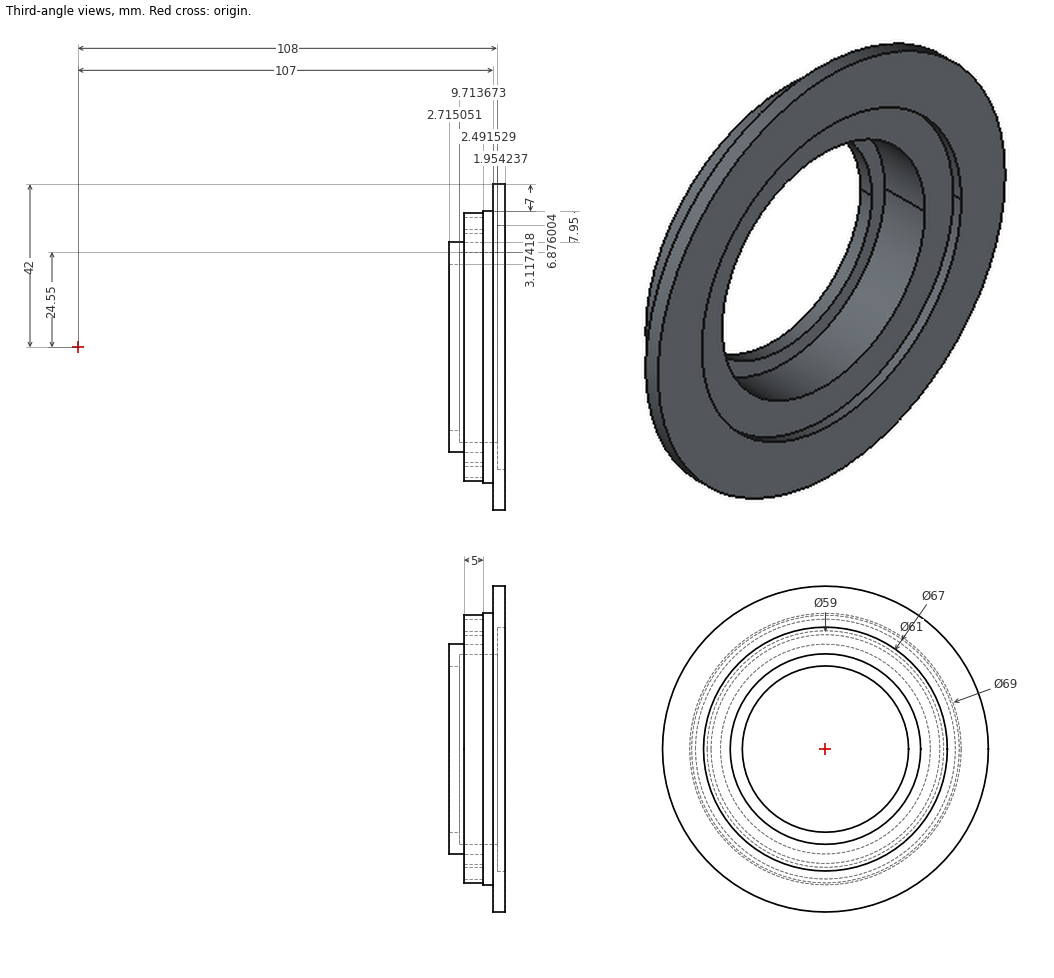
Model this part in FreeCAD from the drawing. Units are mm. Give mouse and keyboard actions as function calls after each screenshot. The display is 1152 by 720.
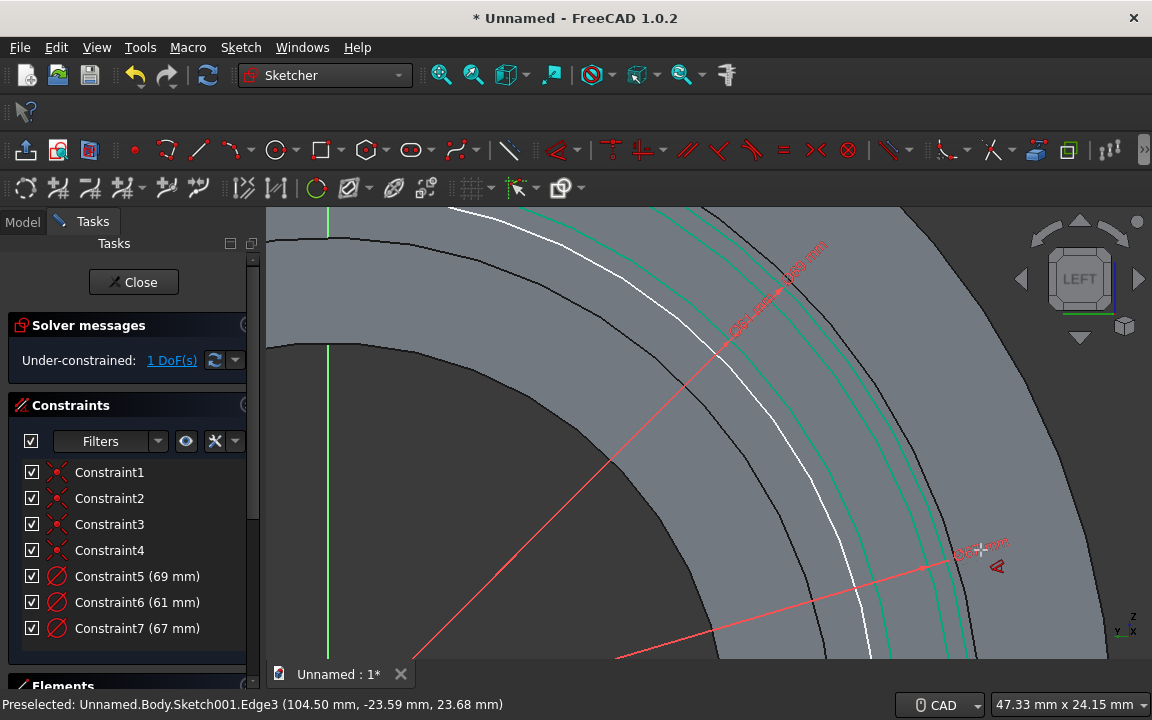
click(716, 353)
click(909, 571)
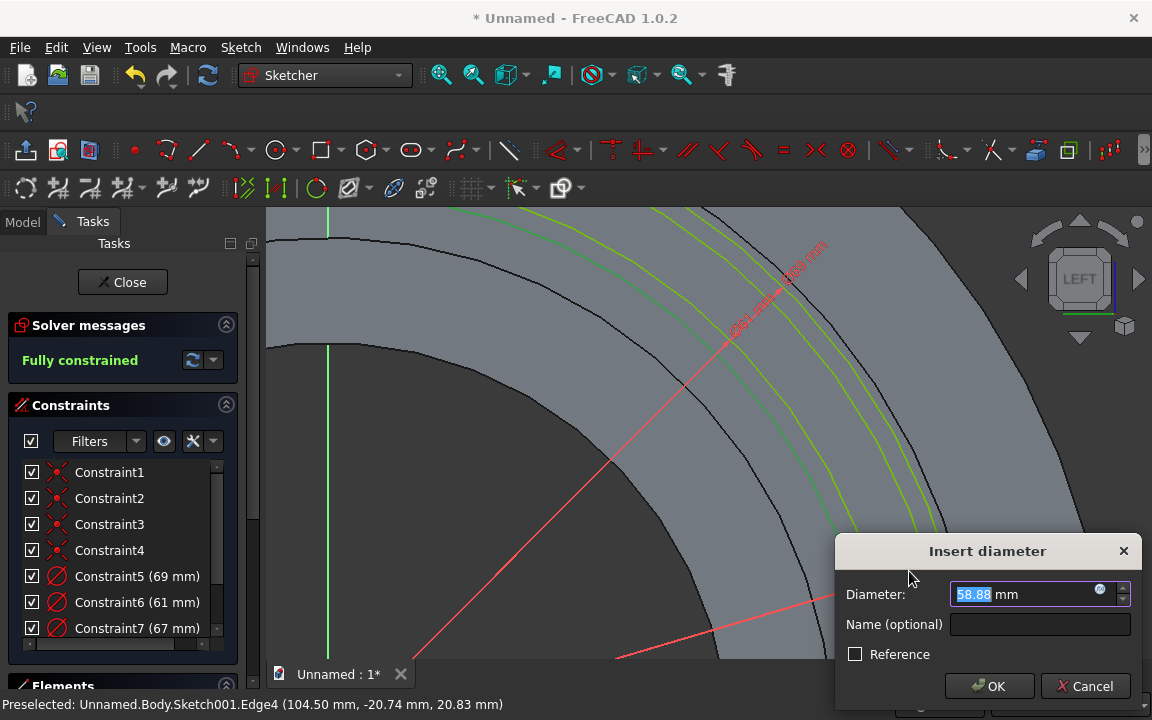
text(59)
key(Return)
key(Escape)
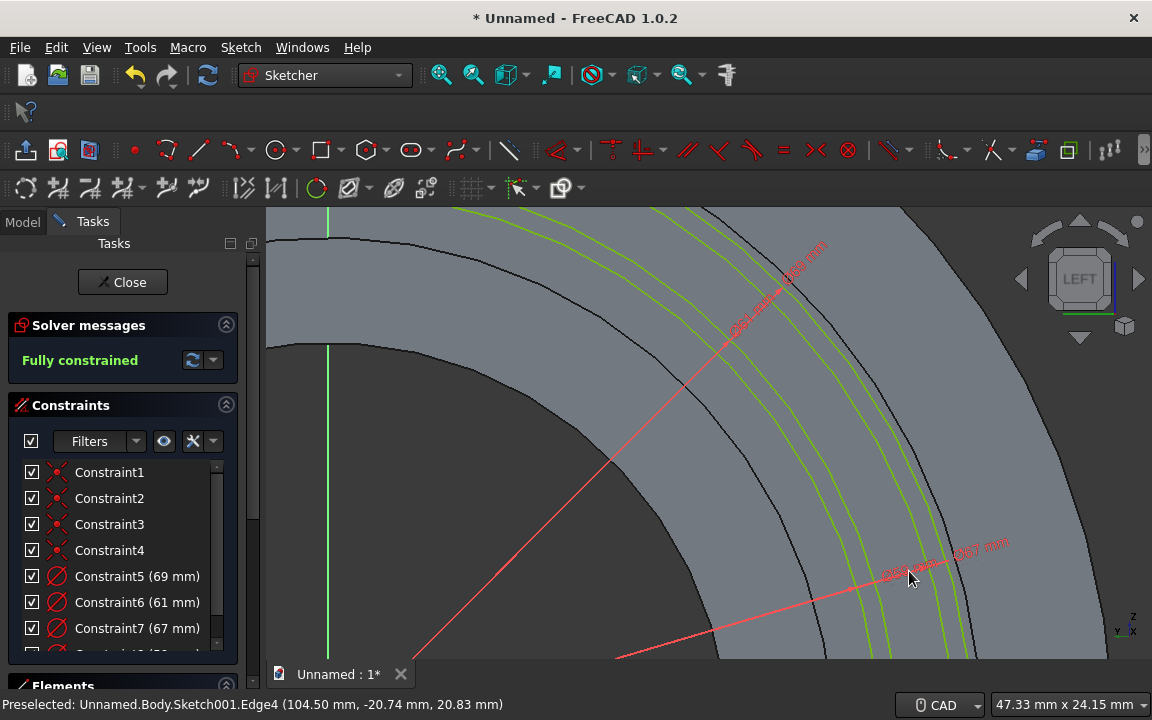
click(123, 282)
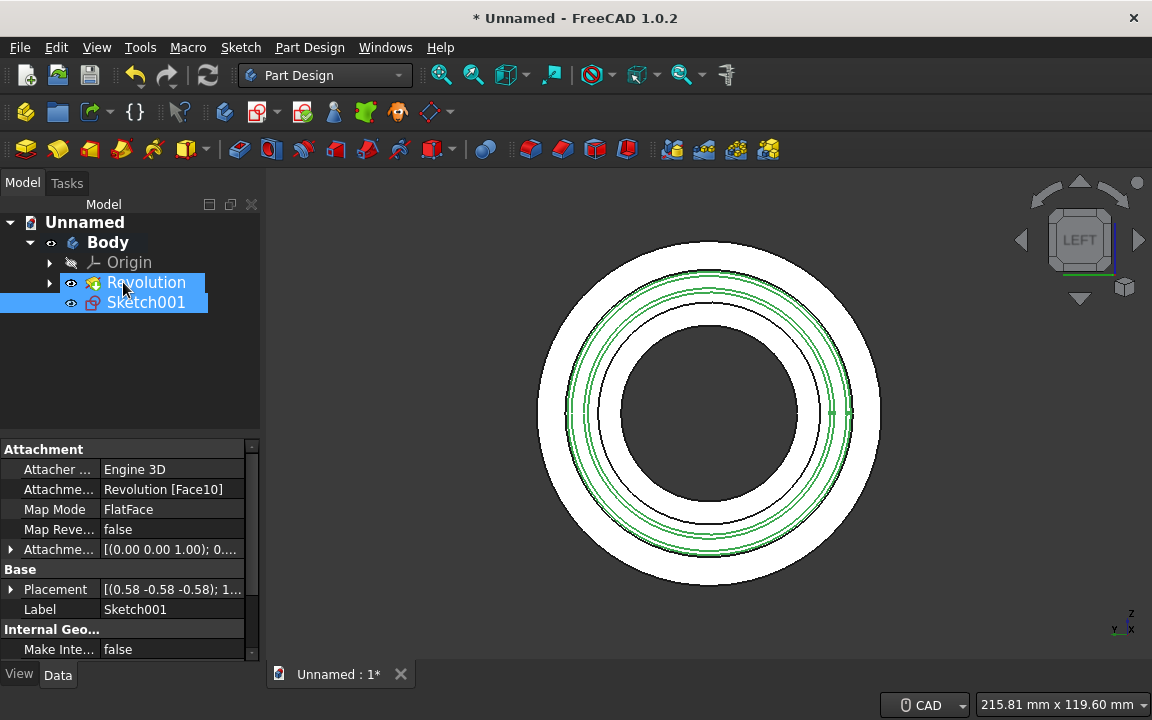
click(26, 150)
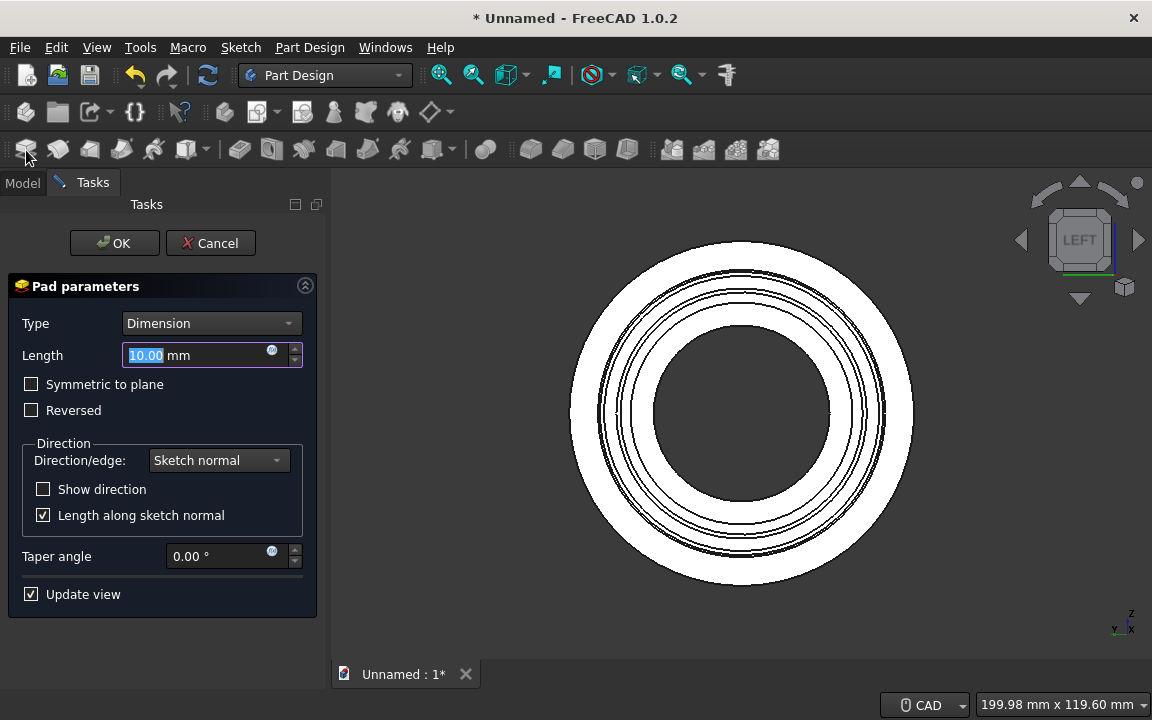
text(5)
key(Tab)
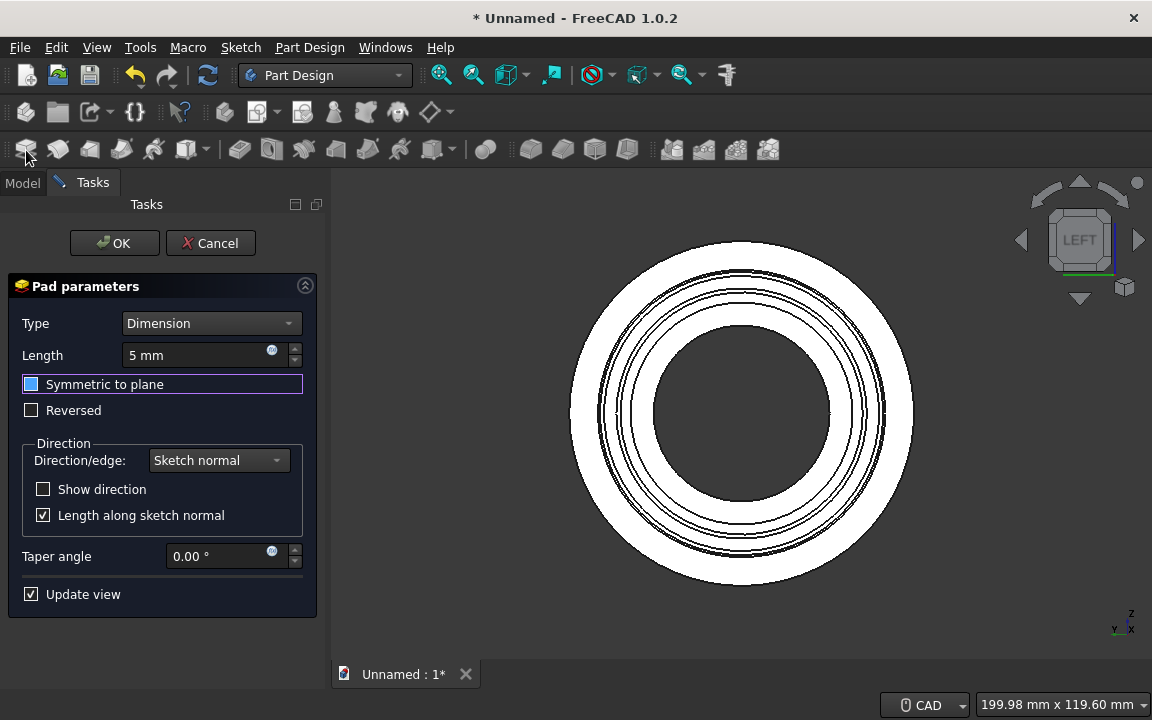
click(115, 243)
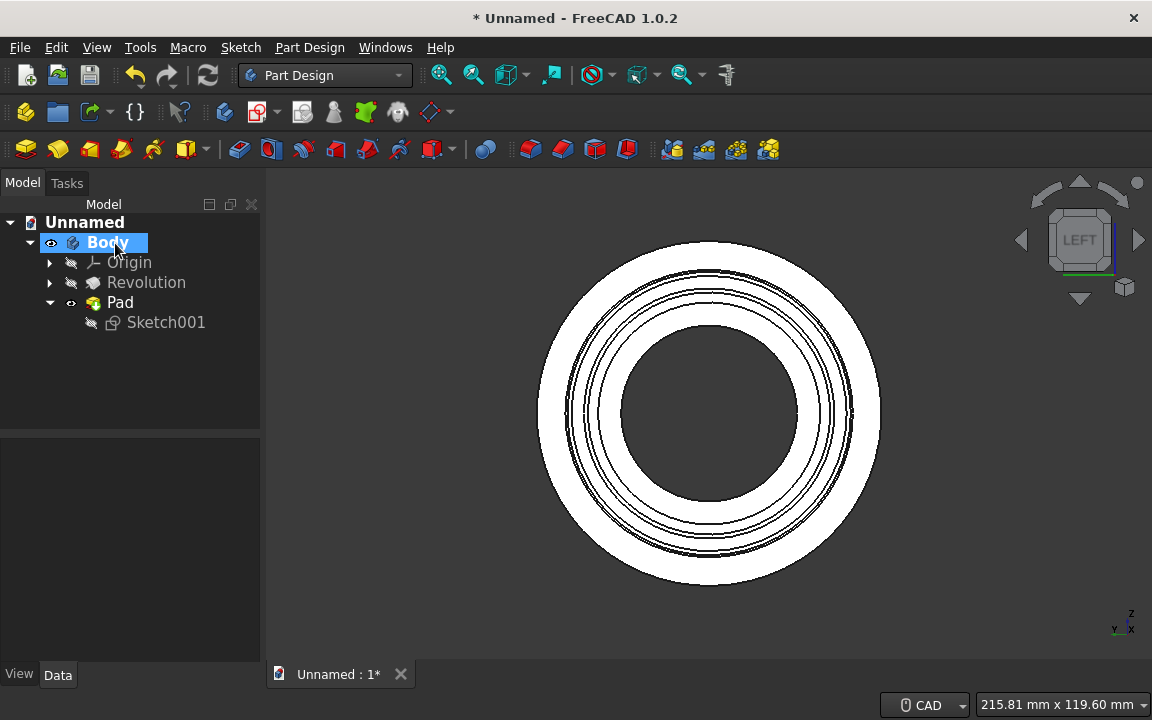
key(0)